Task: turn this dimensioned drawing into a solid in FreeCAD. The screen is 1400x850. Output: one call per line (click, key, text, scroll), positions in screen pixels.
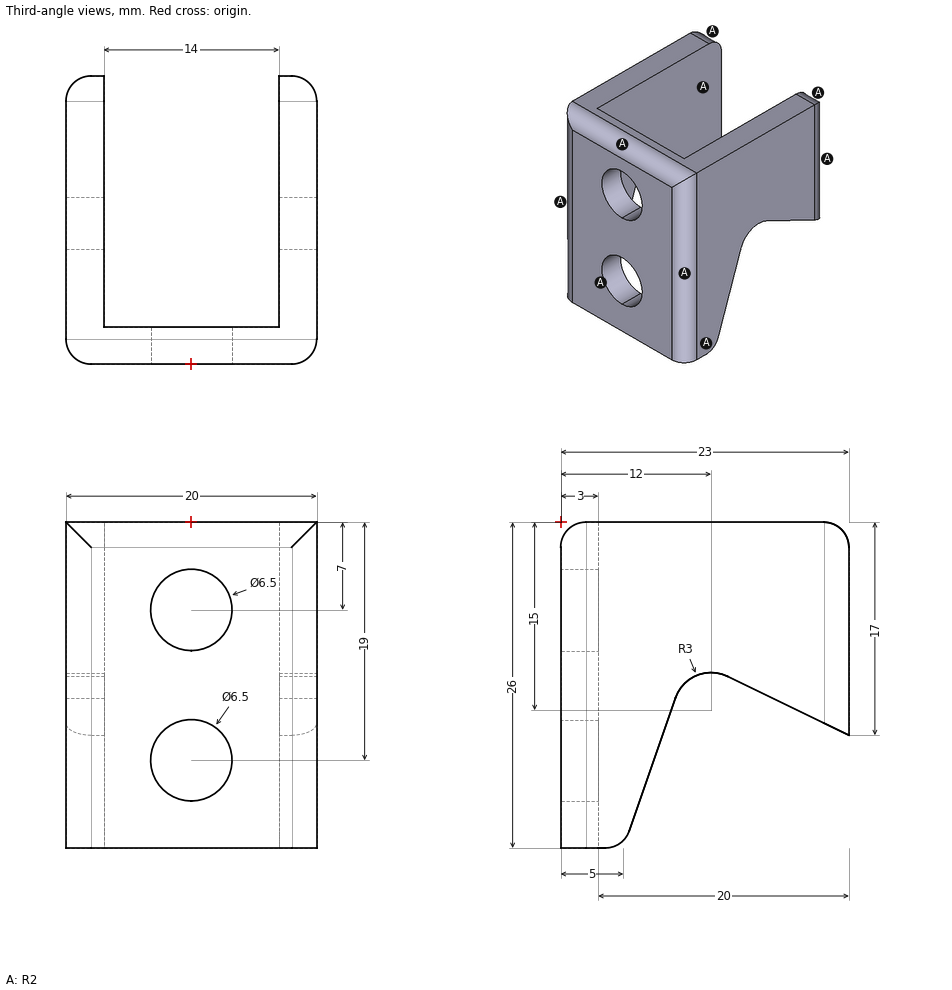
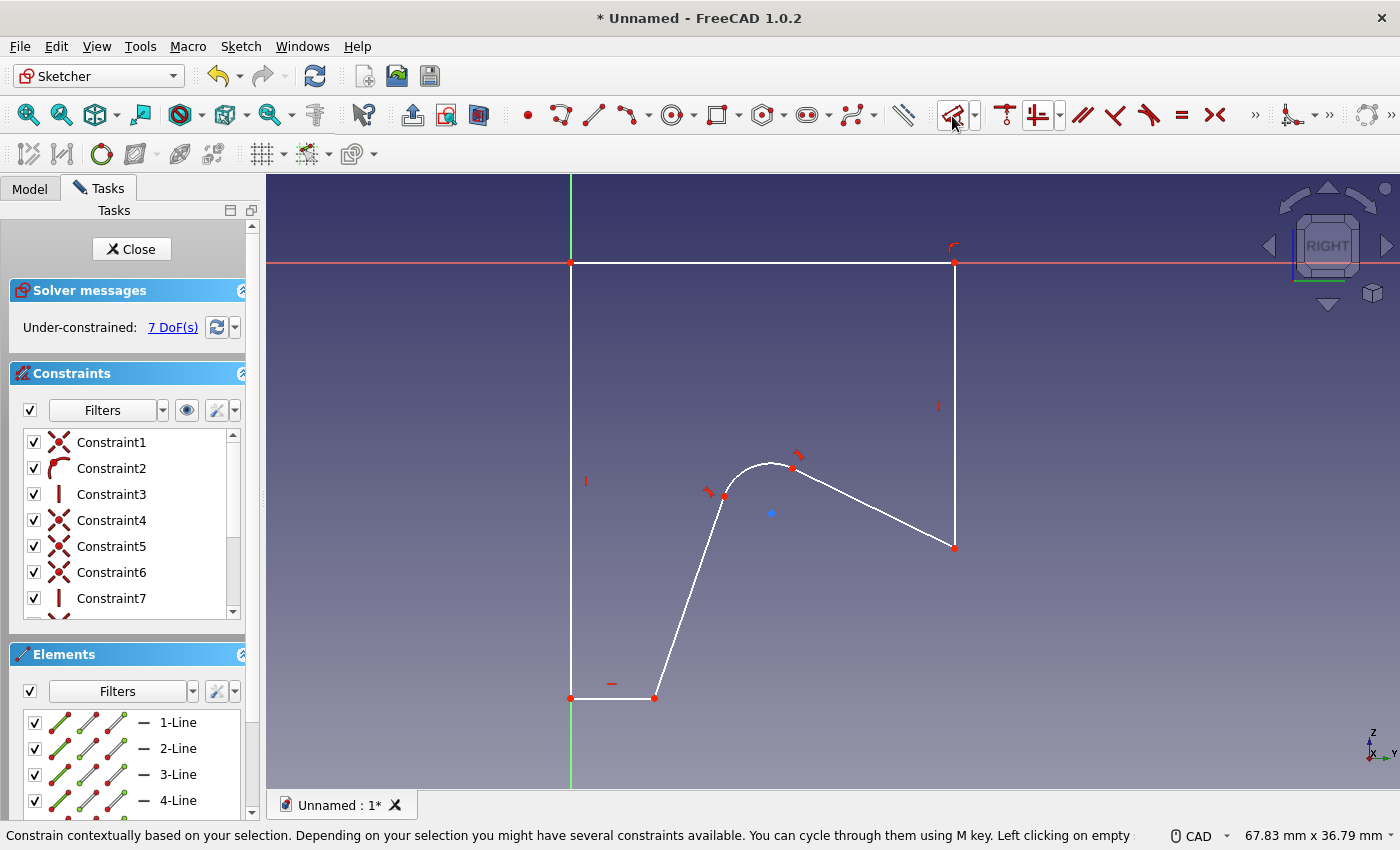
click(768, 463)
click(766, 431)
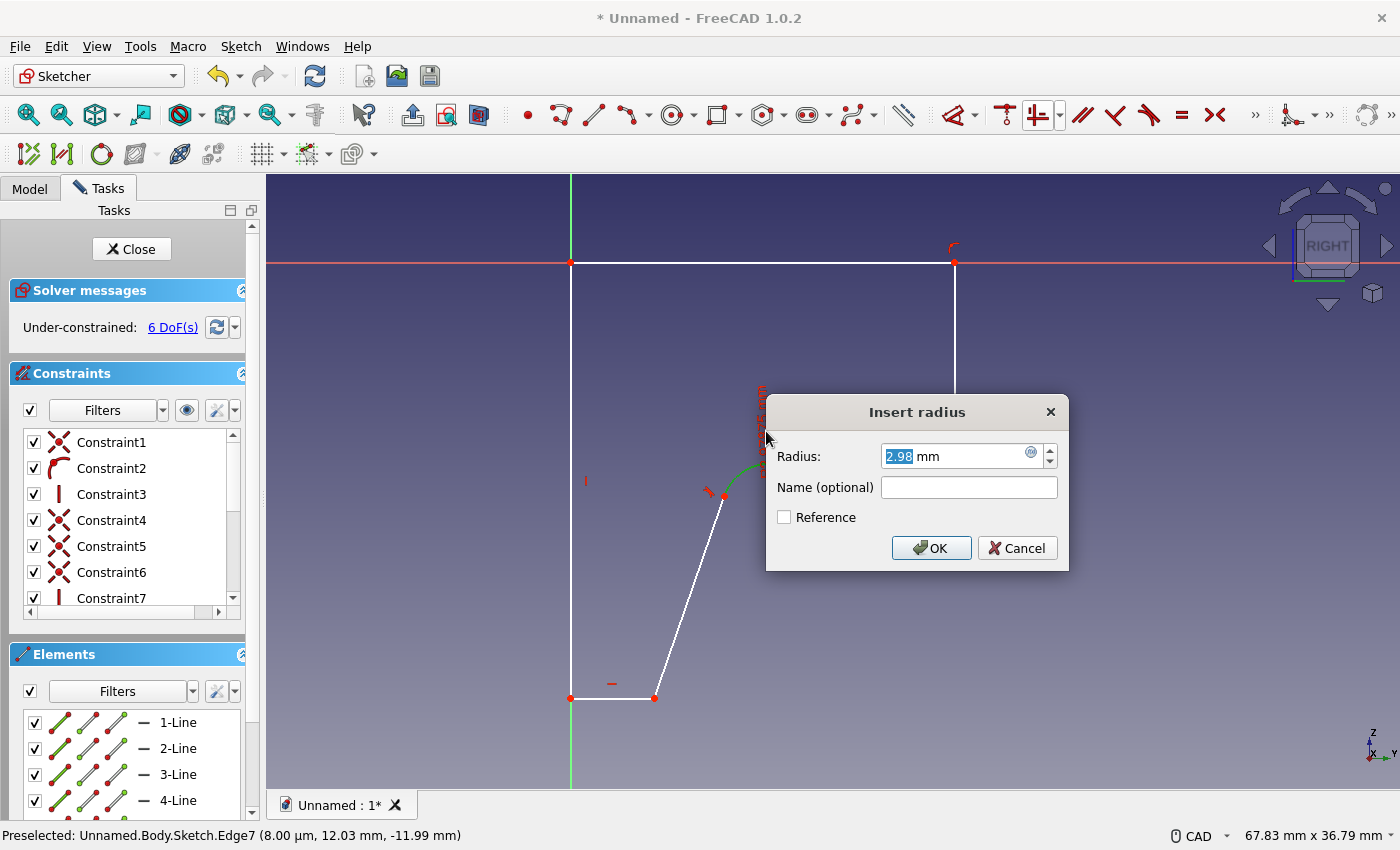
text(3)
key(Return)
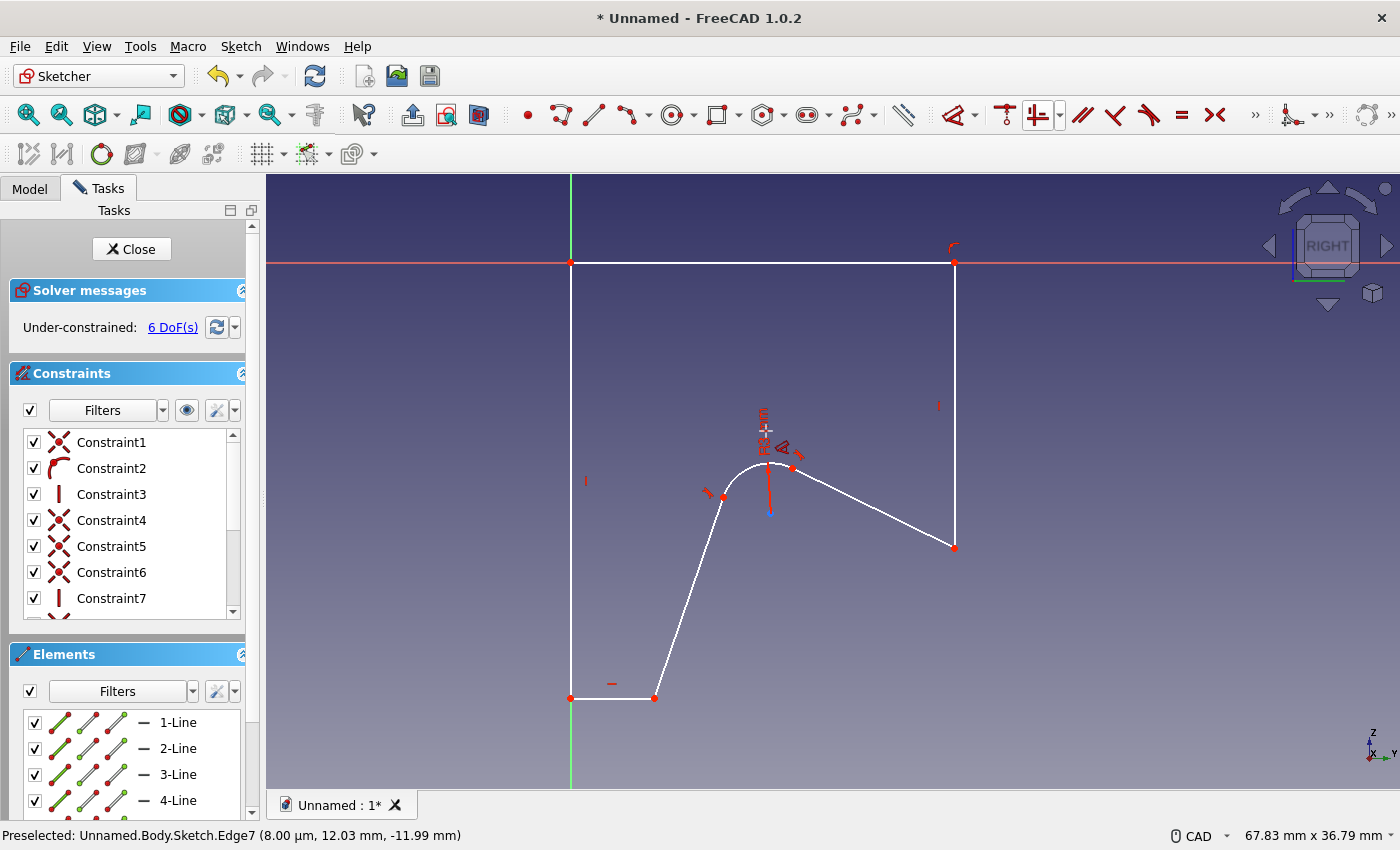
click(596, 699)
click(612, 733)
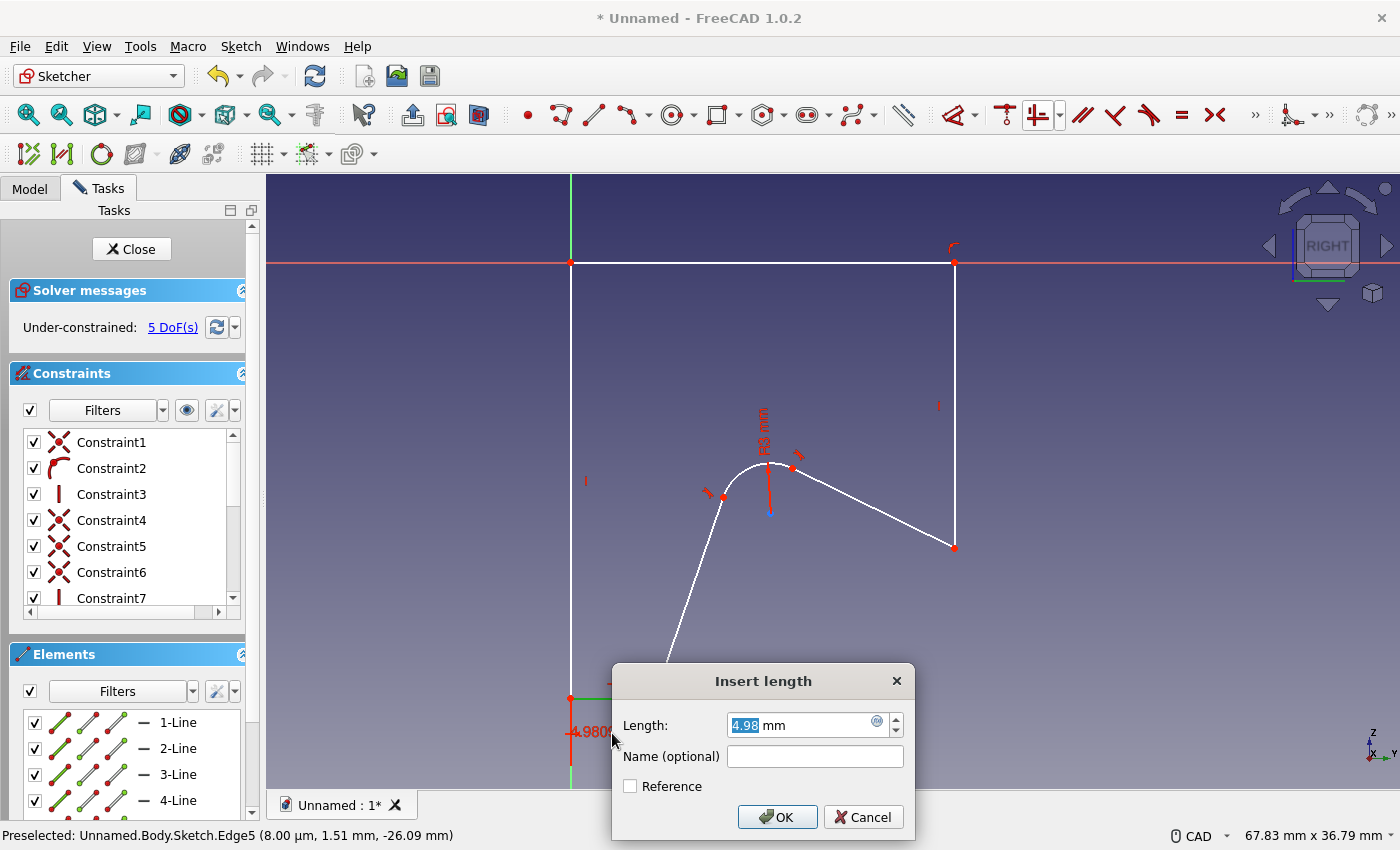
text(5)
key(Return)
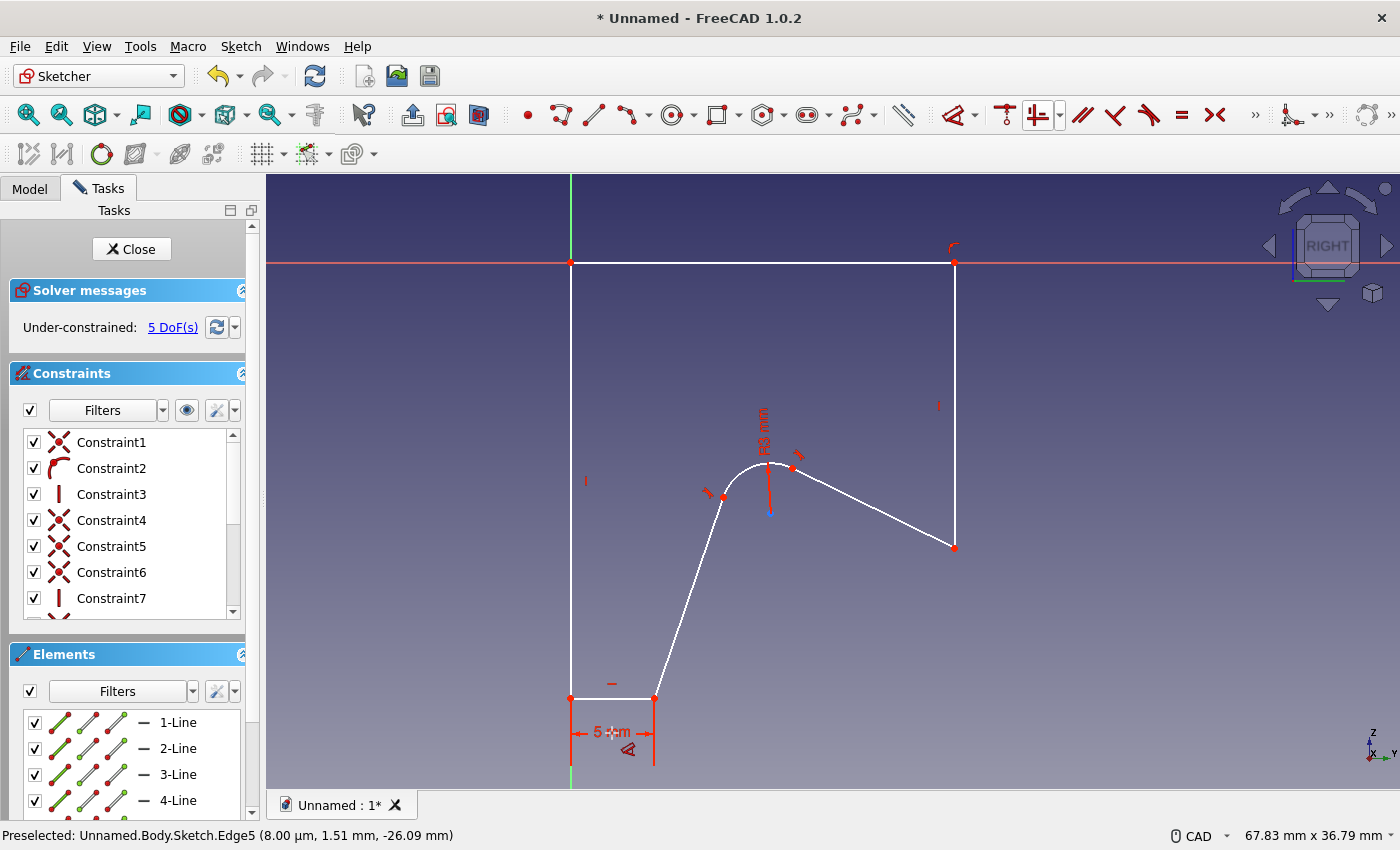
click(955, 462)
click(989, 405)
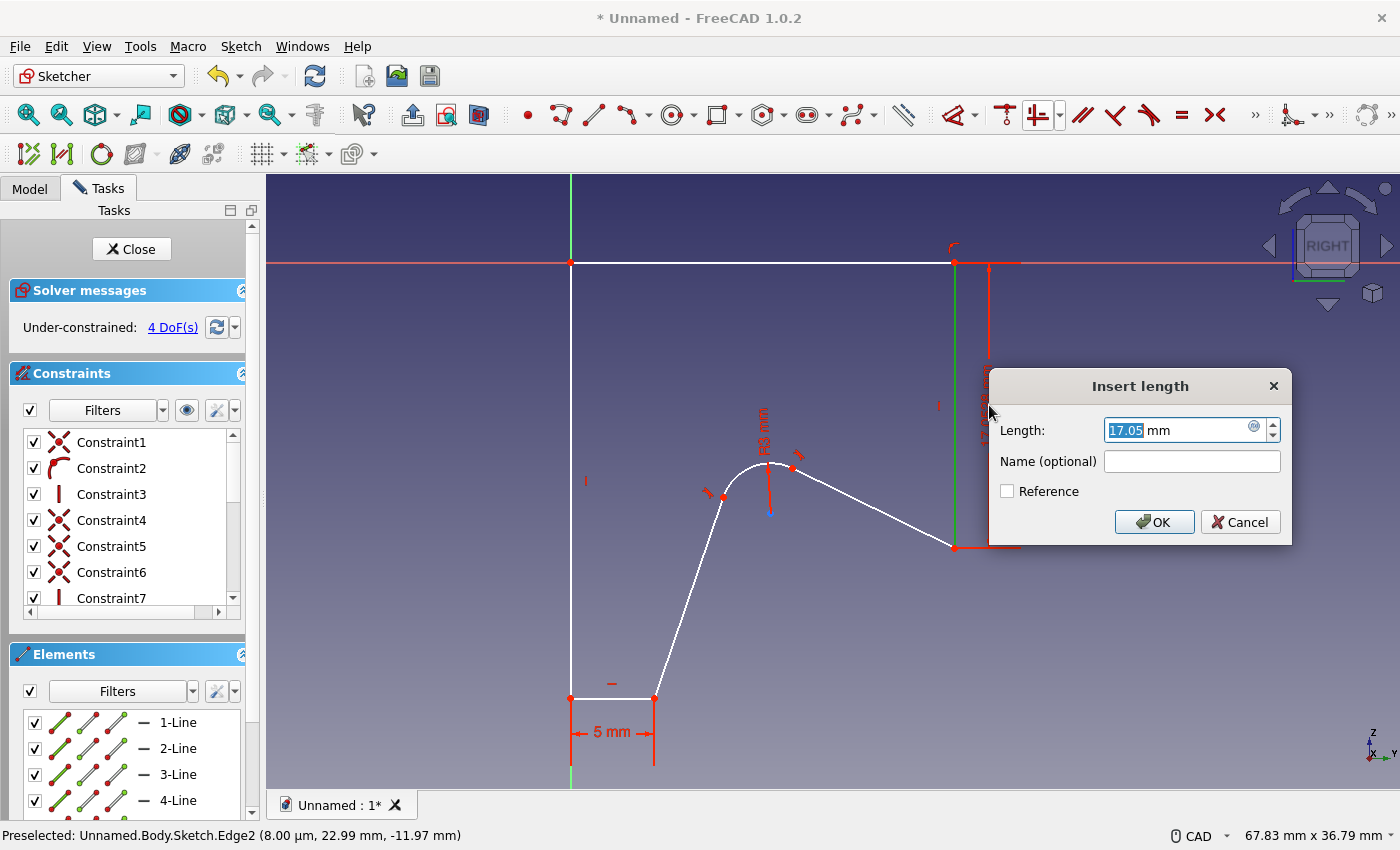
text(17)
key(Return)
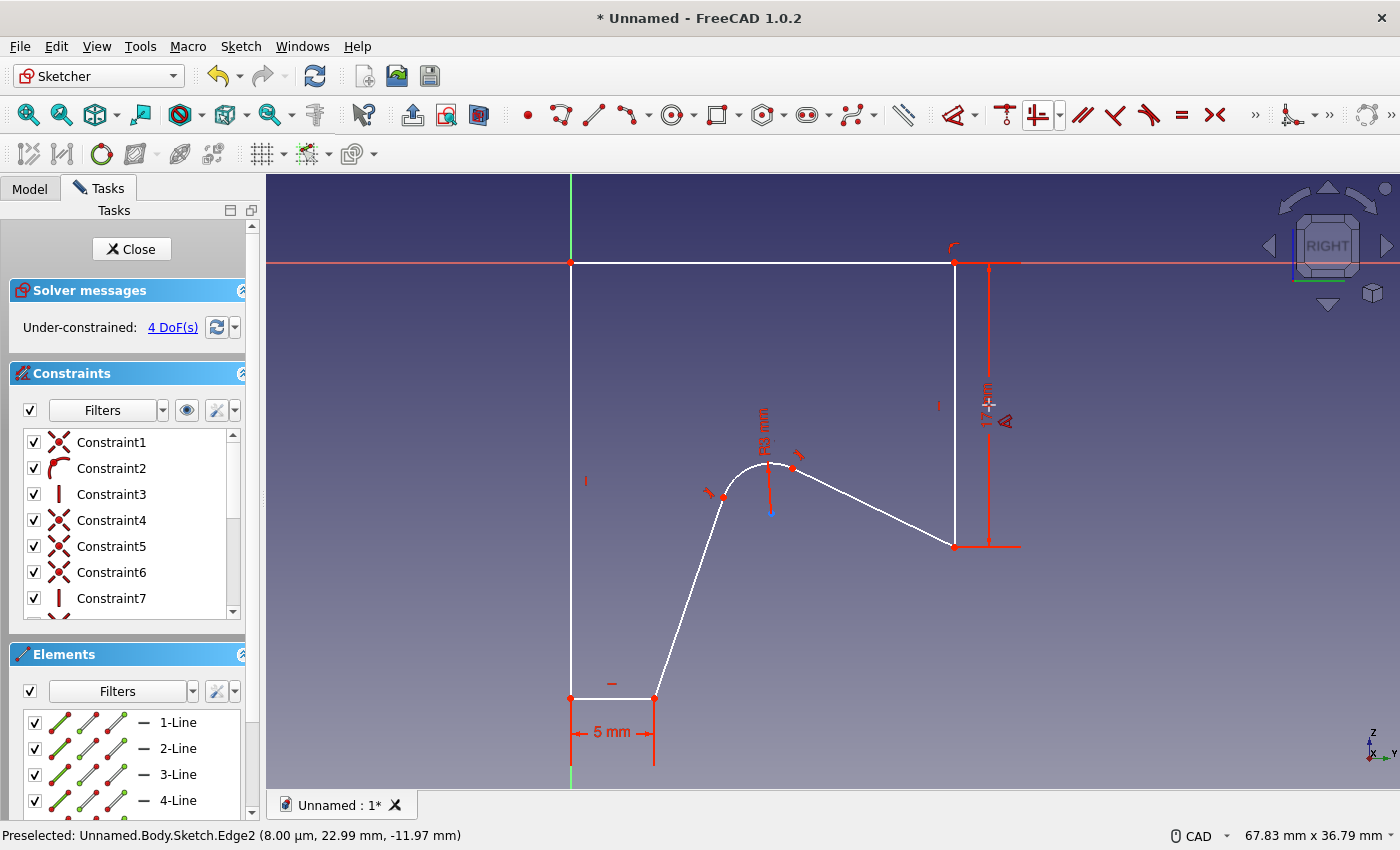
click(840, 263)
click(763, 229)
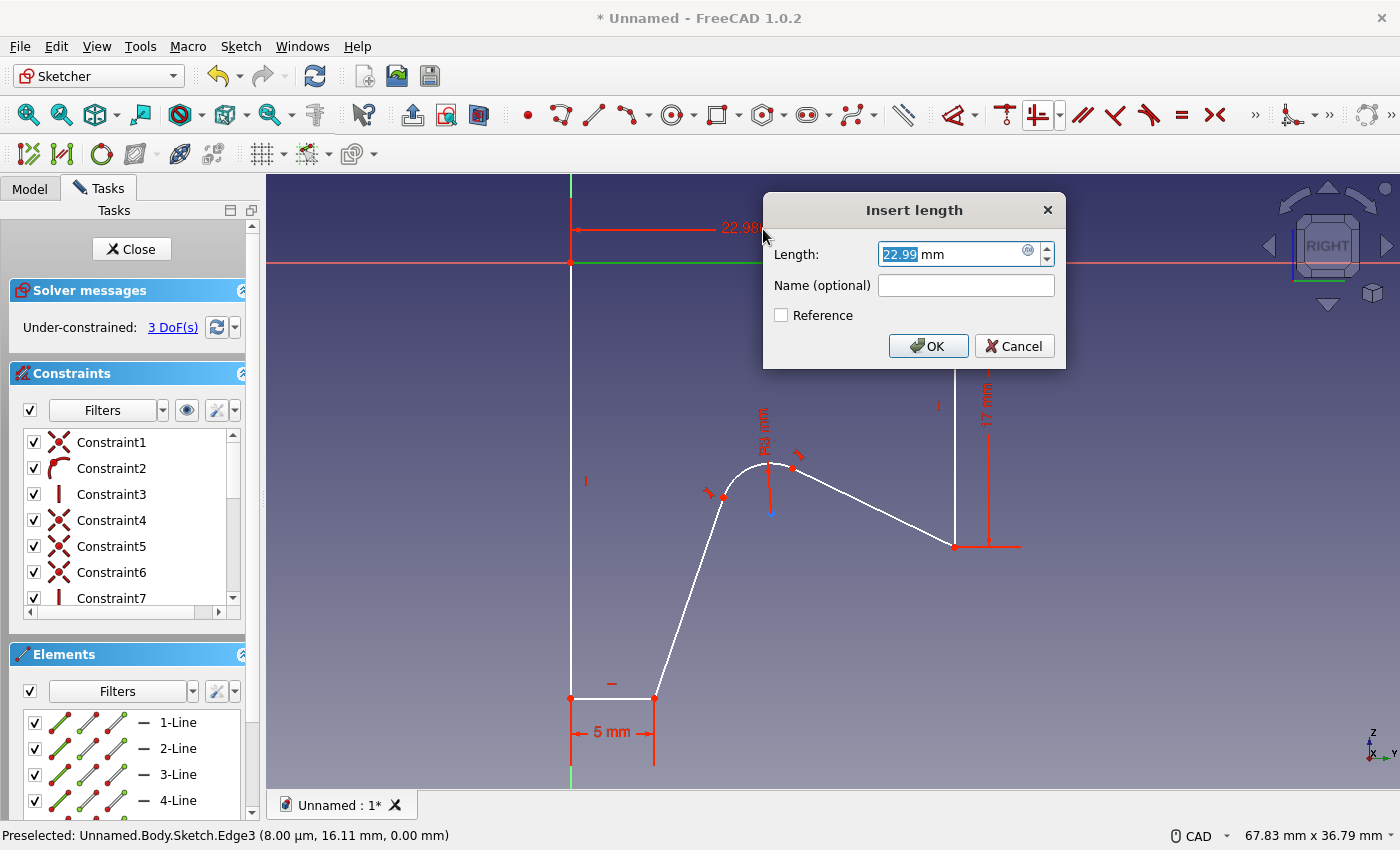
text(23)
key(Return)